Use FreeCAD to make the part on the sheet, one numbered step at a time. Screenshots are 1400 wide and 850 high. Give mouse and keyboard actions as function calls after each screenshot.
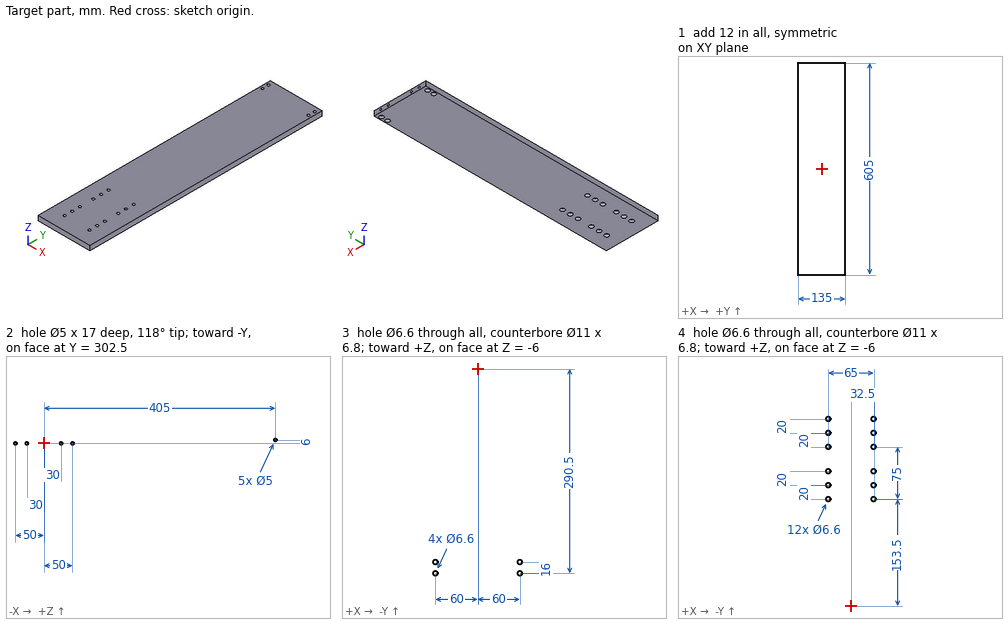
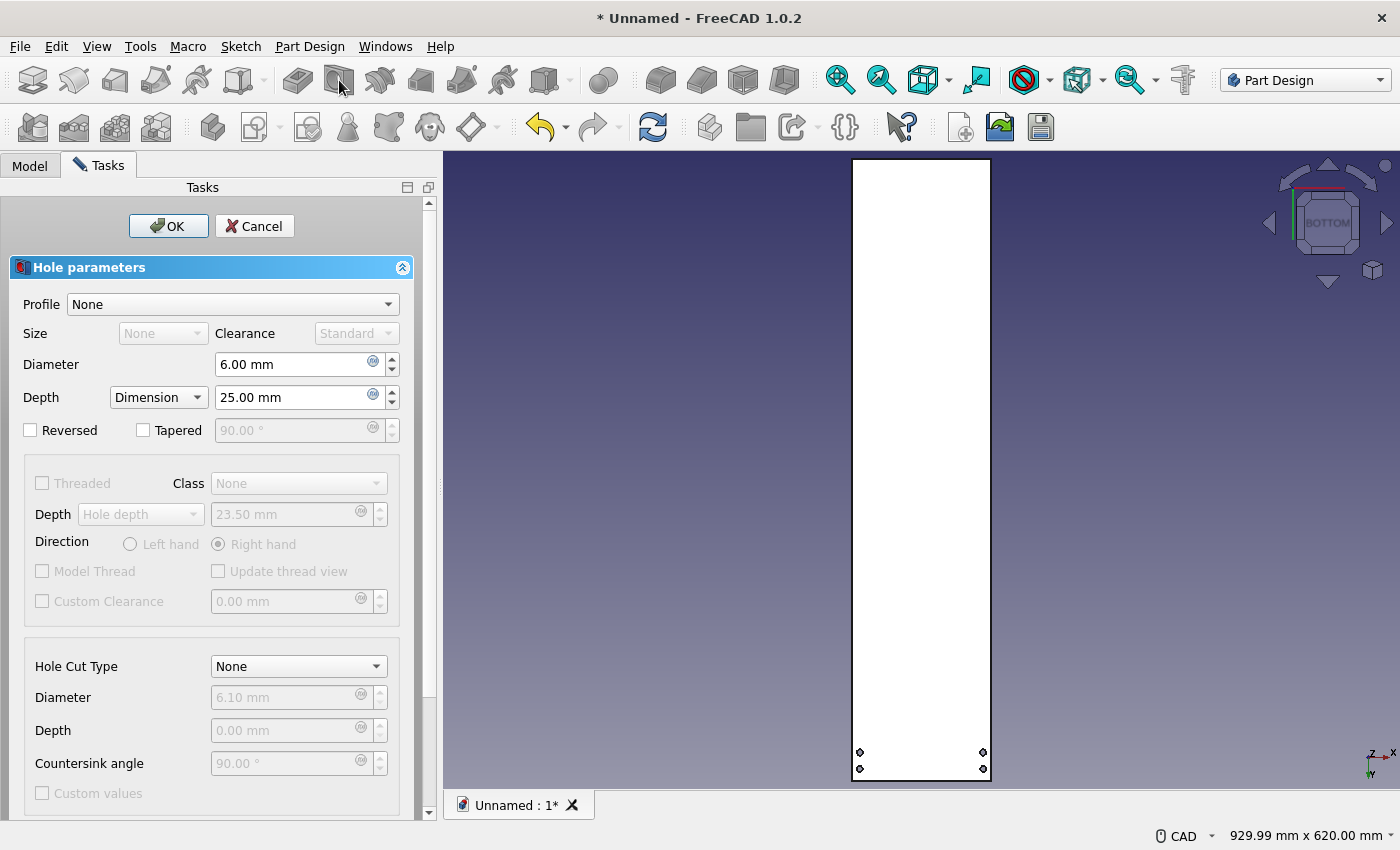
triple_click(300, 364)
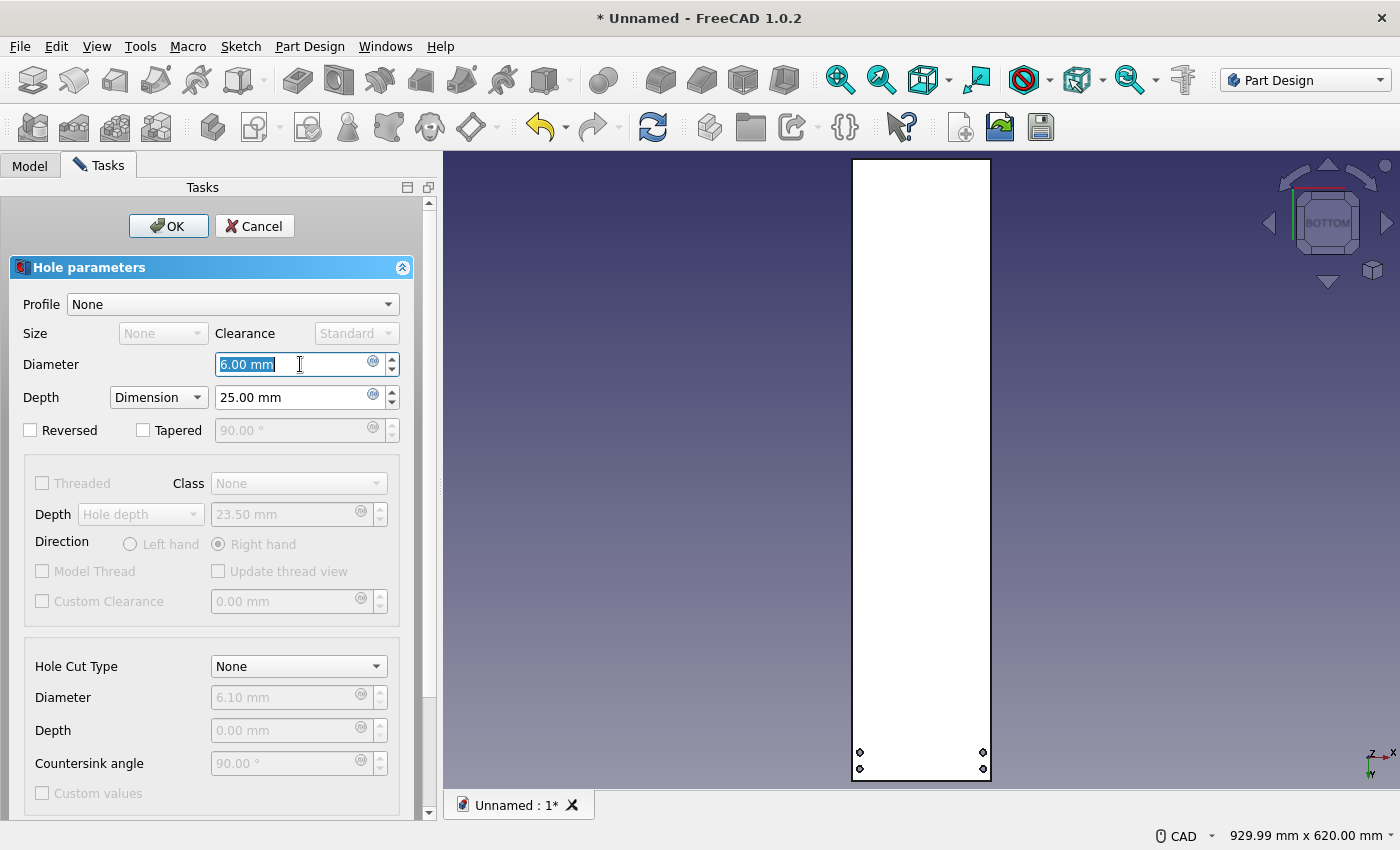
text(6.6)
key(Tab)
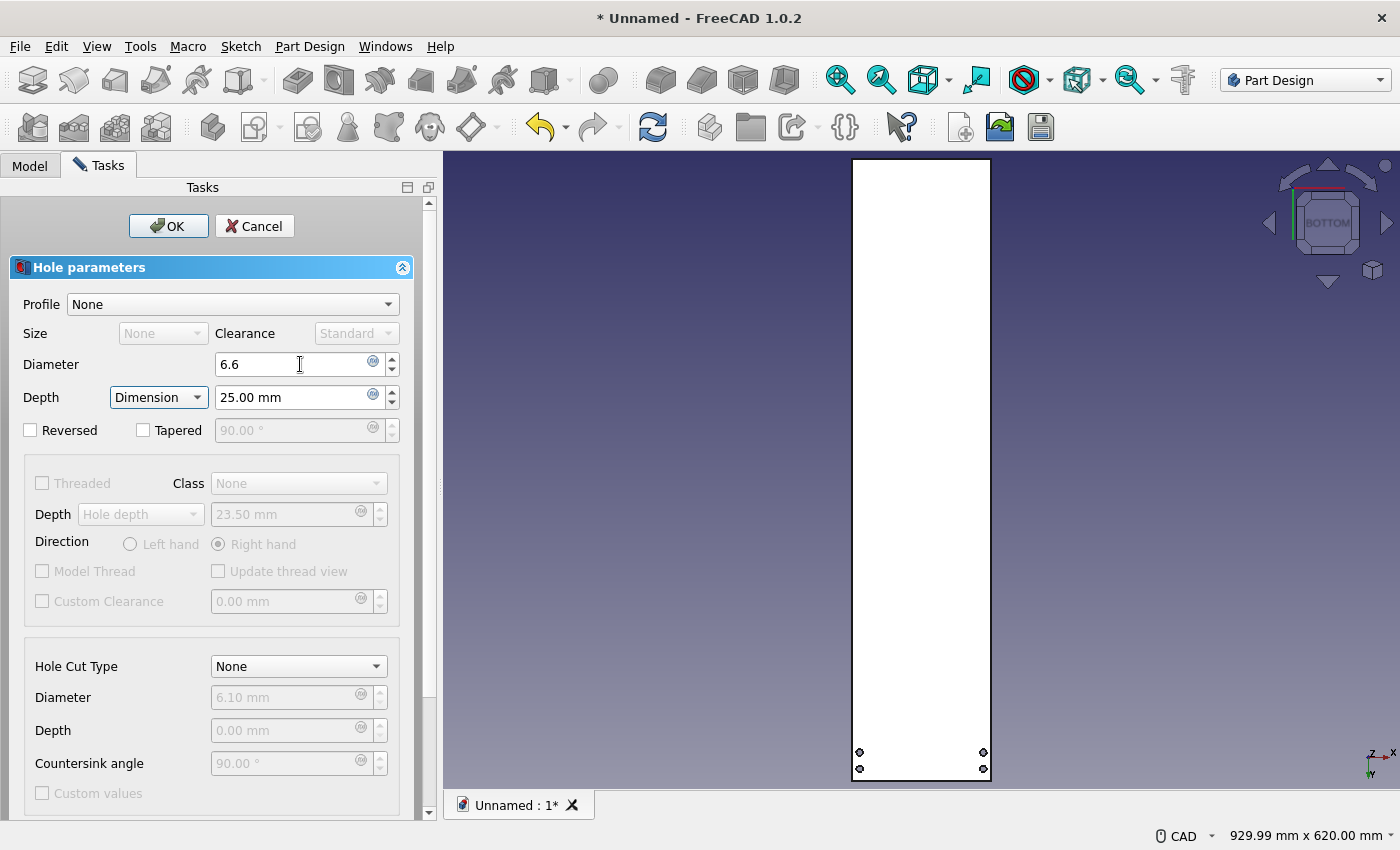
click(160, 398)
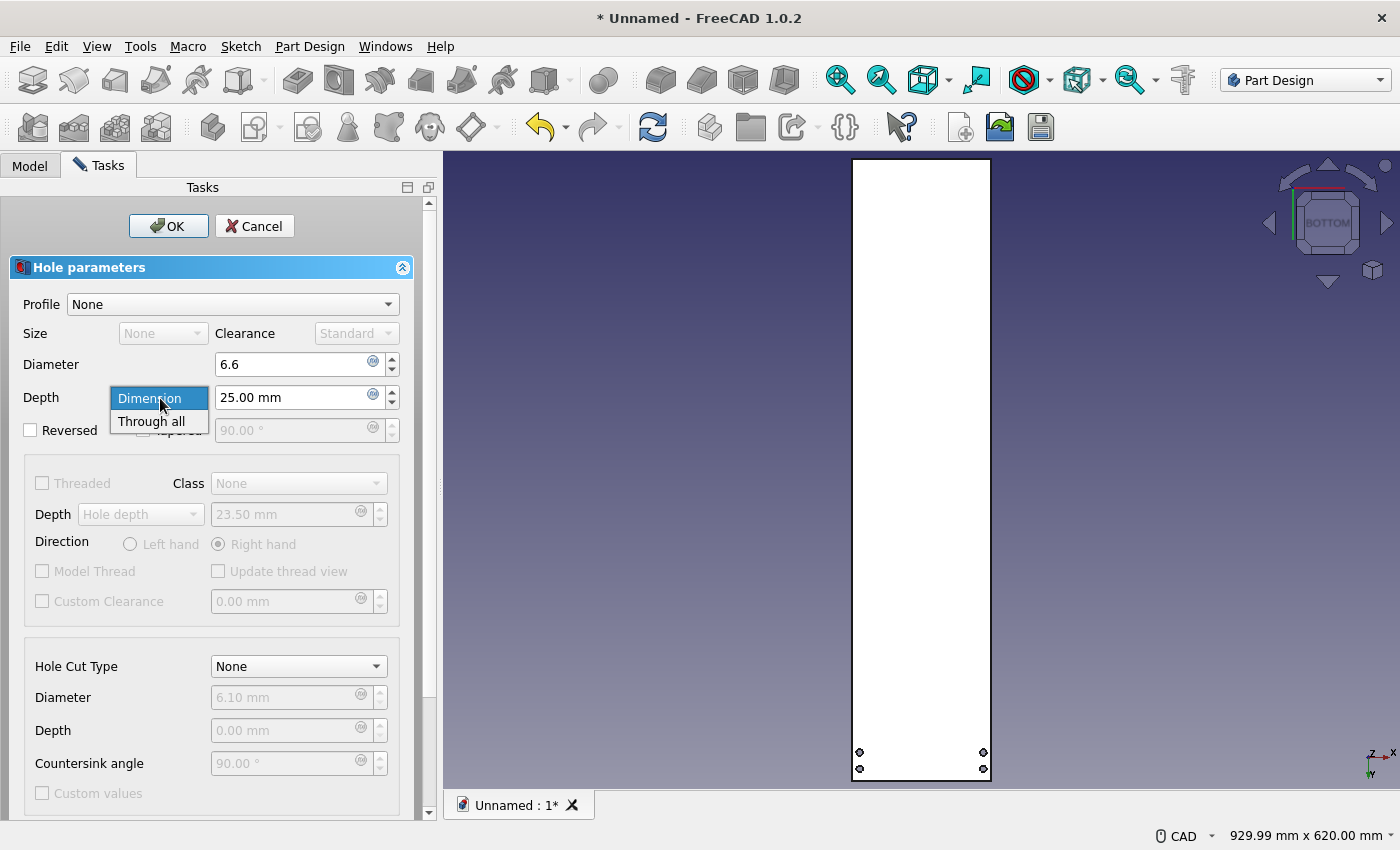
click(158, 422)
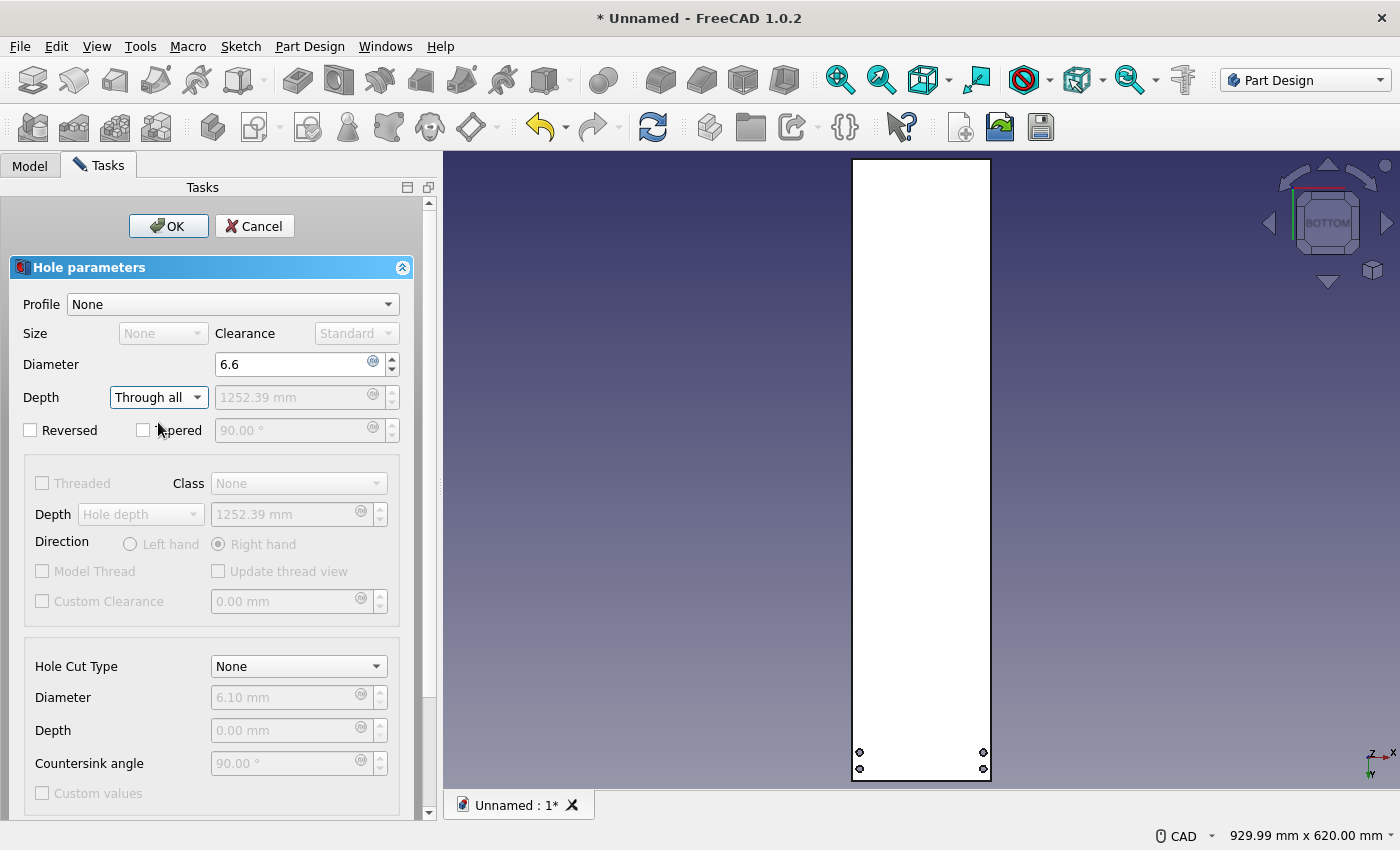
click(300, 666)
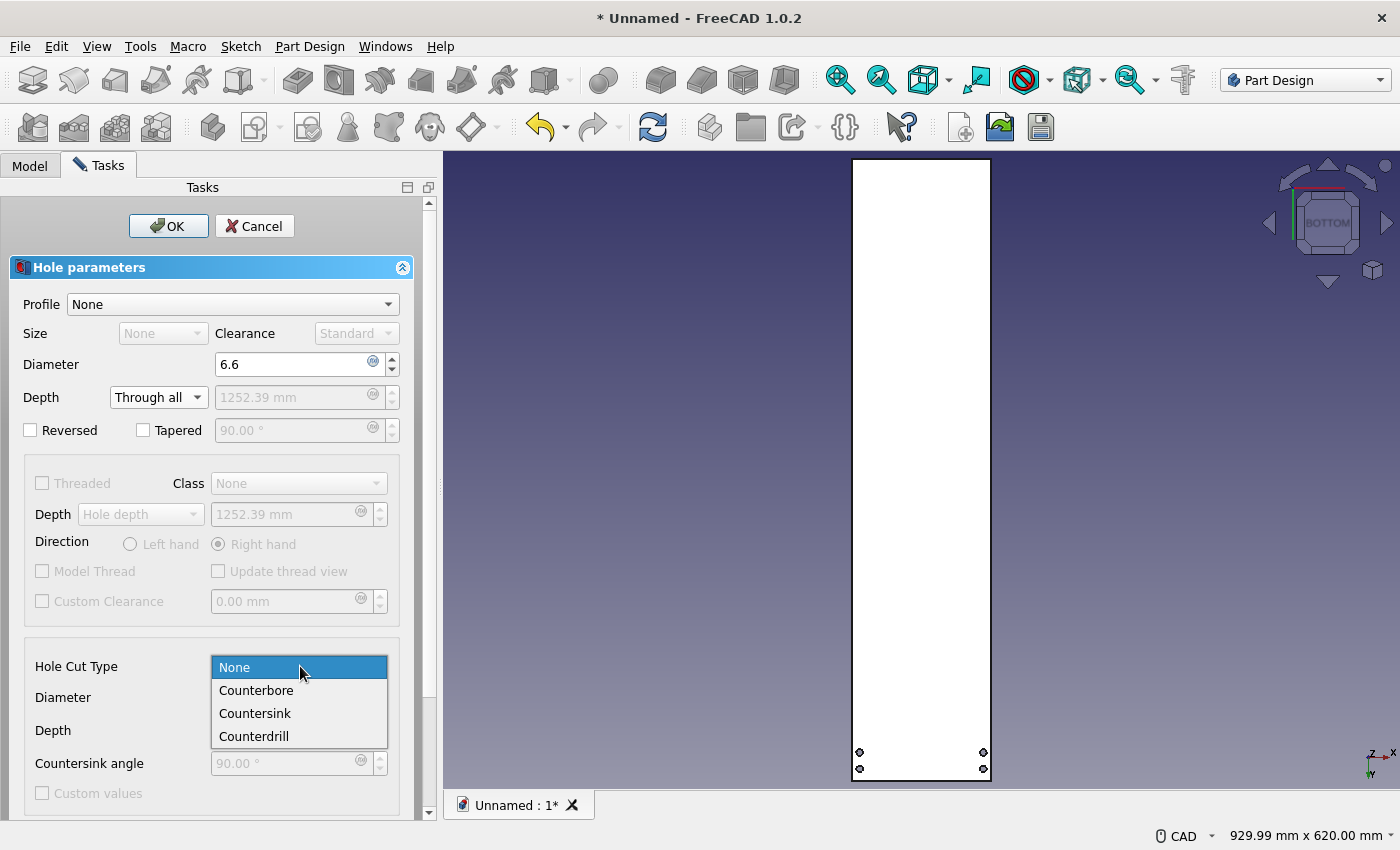
click(298, 690)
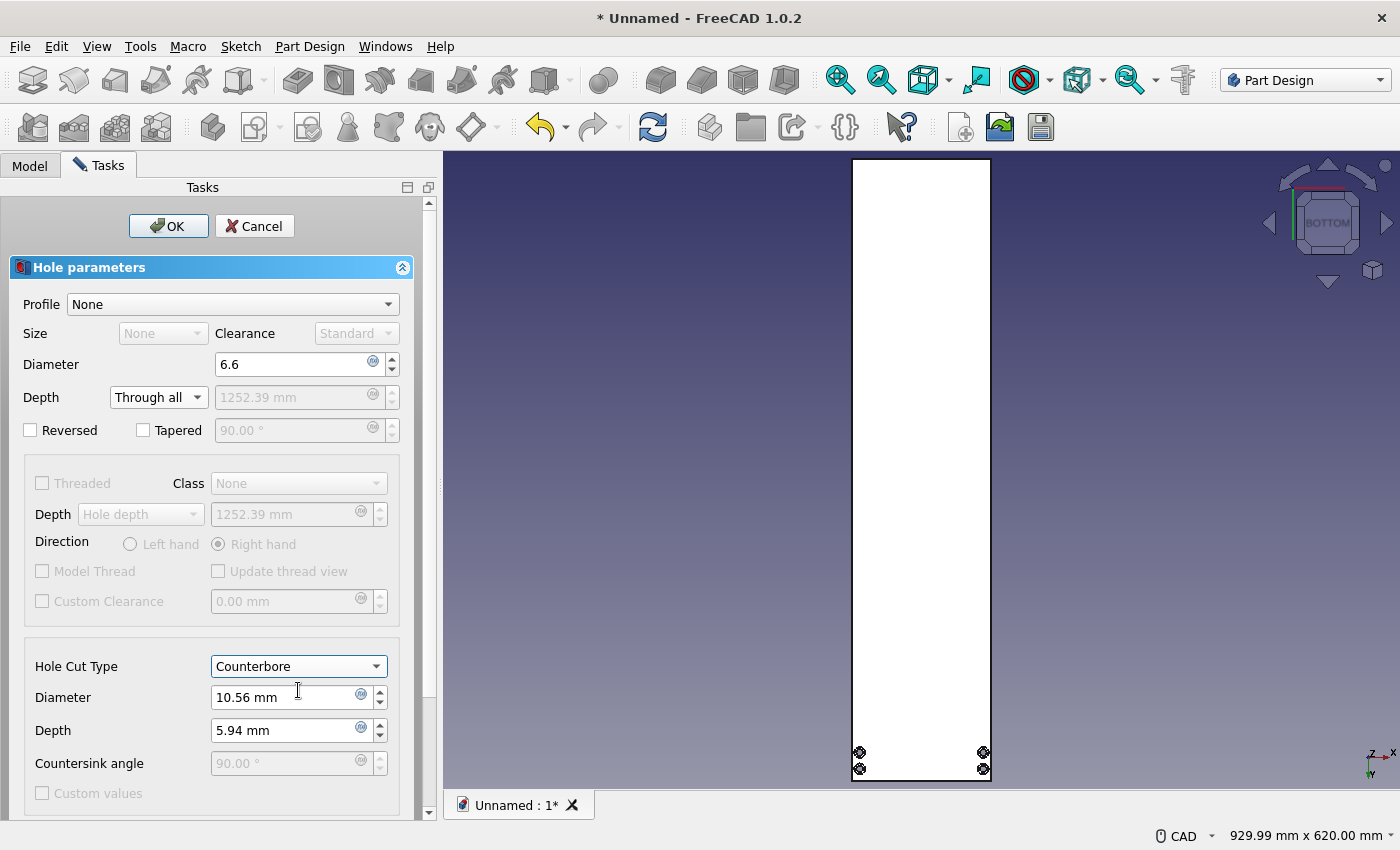
triple_click(292, 698)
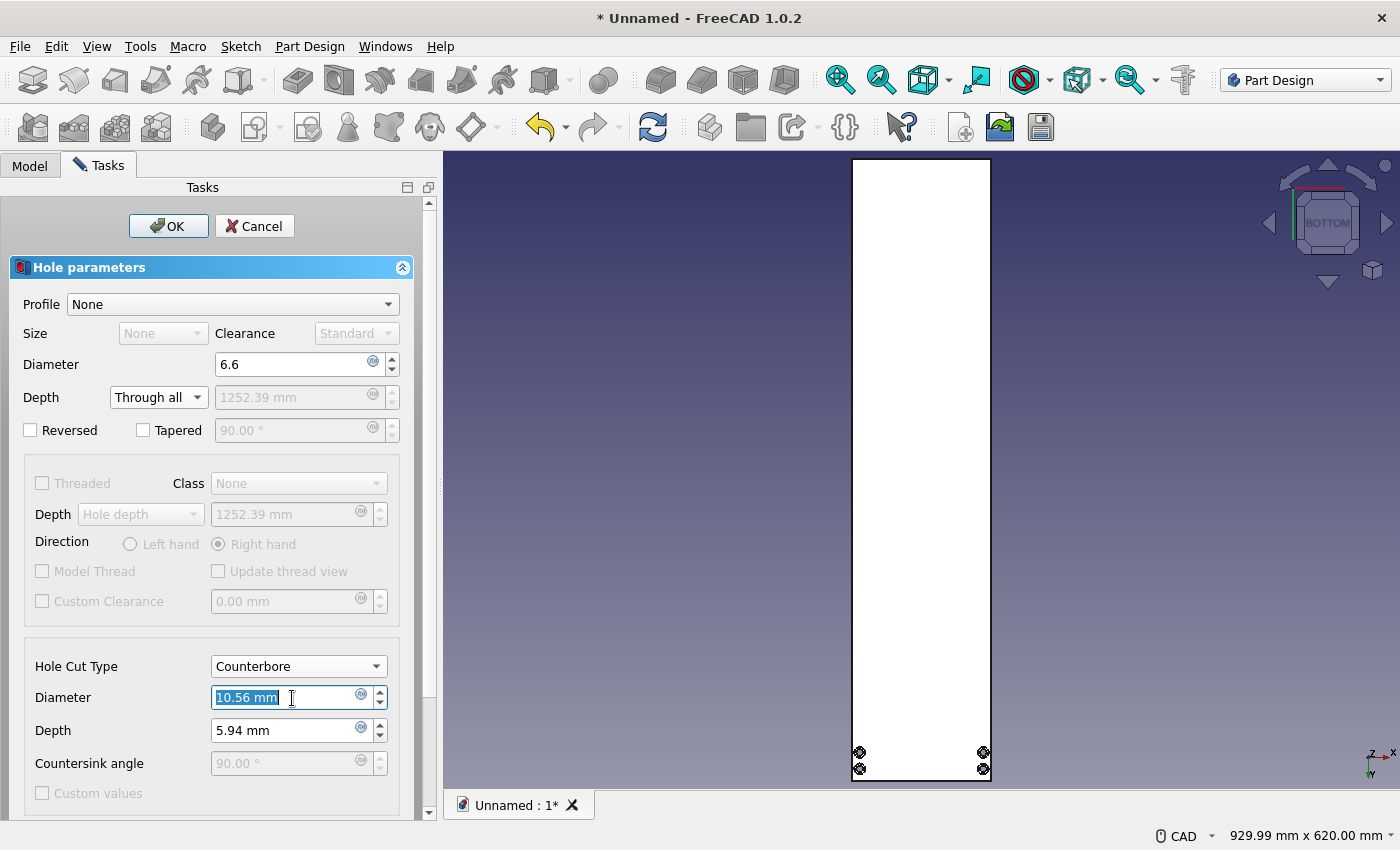
text(11)
key(Tab)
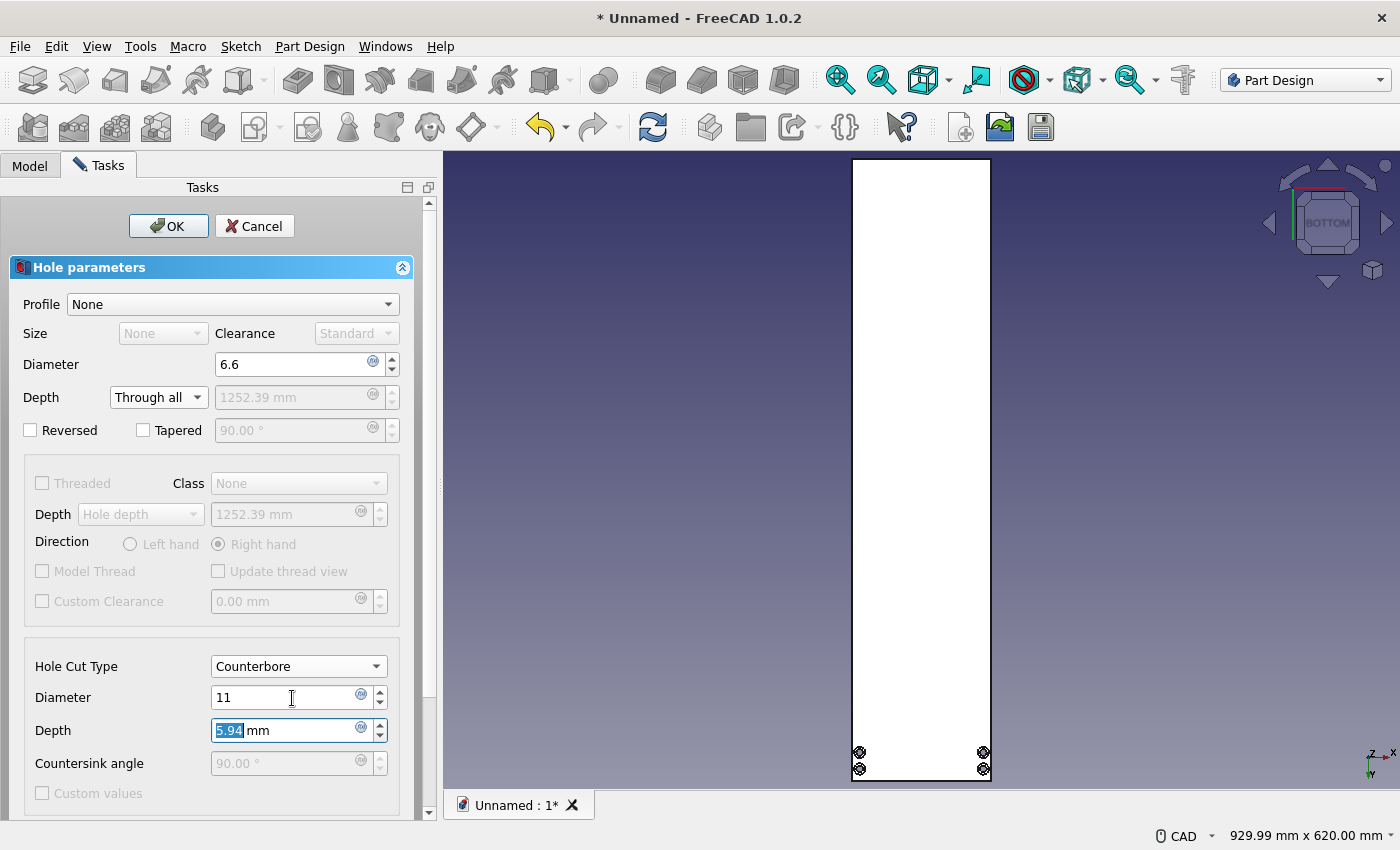
text(6.8)
key(Tab)